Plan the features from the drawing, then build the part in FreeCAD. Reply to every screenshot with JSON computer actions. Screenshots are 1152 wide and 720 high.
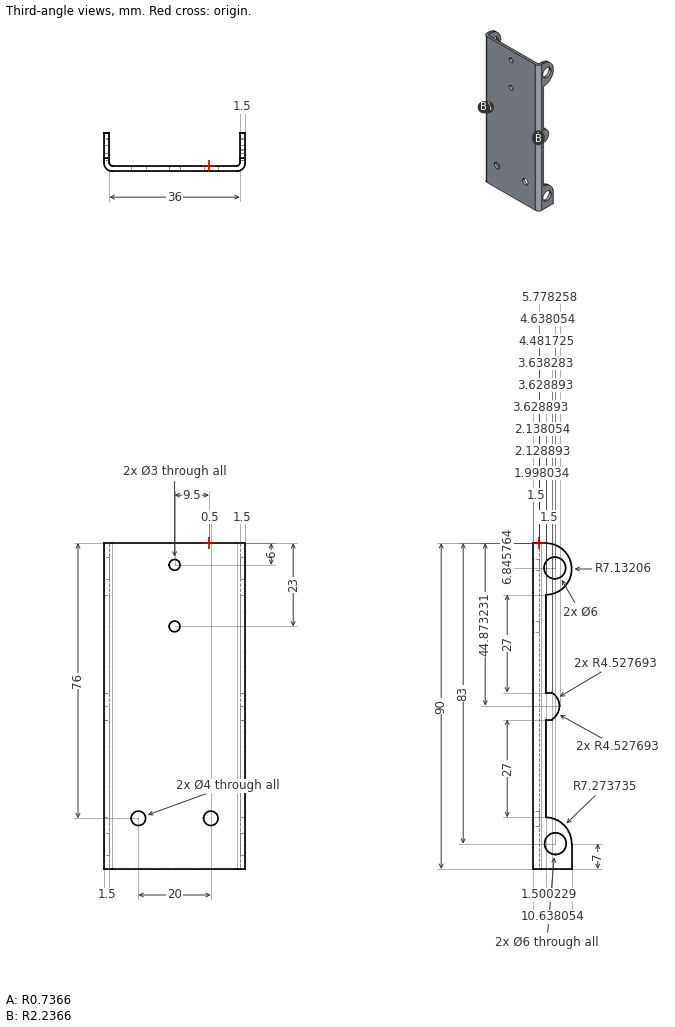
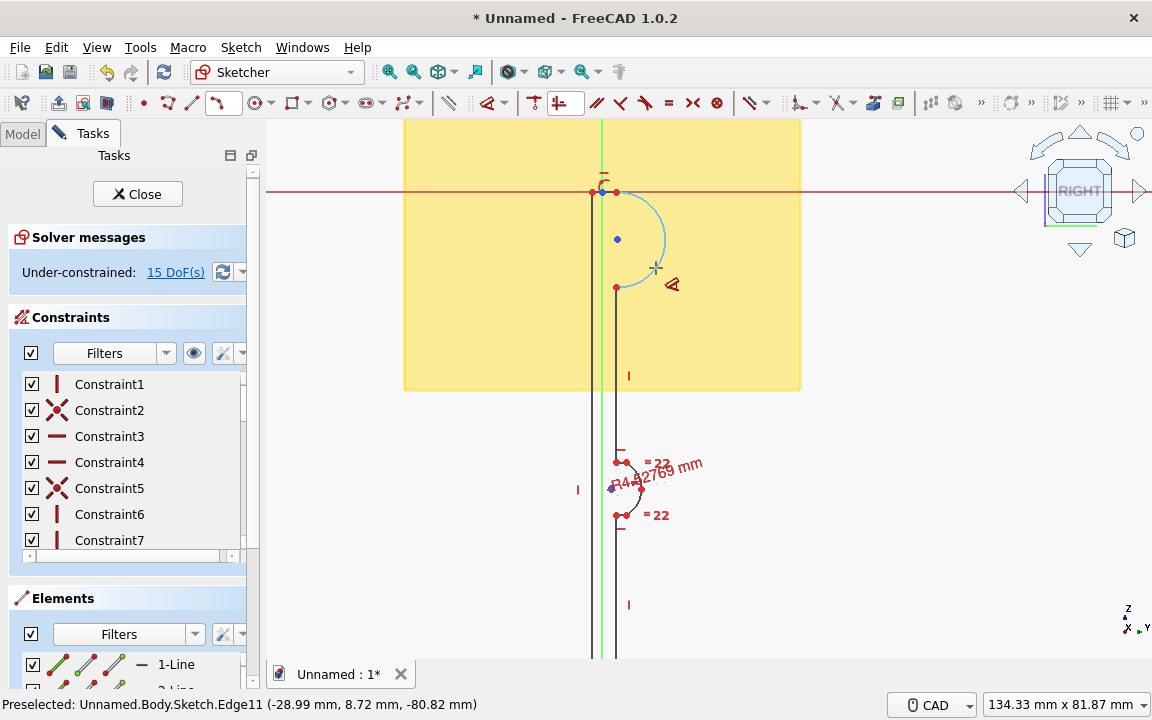
{"action": "left_click", "coordinate": [656, 268]}
{"action": "left_click", "coordinate": [682, 287]}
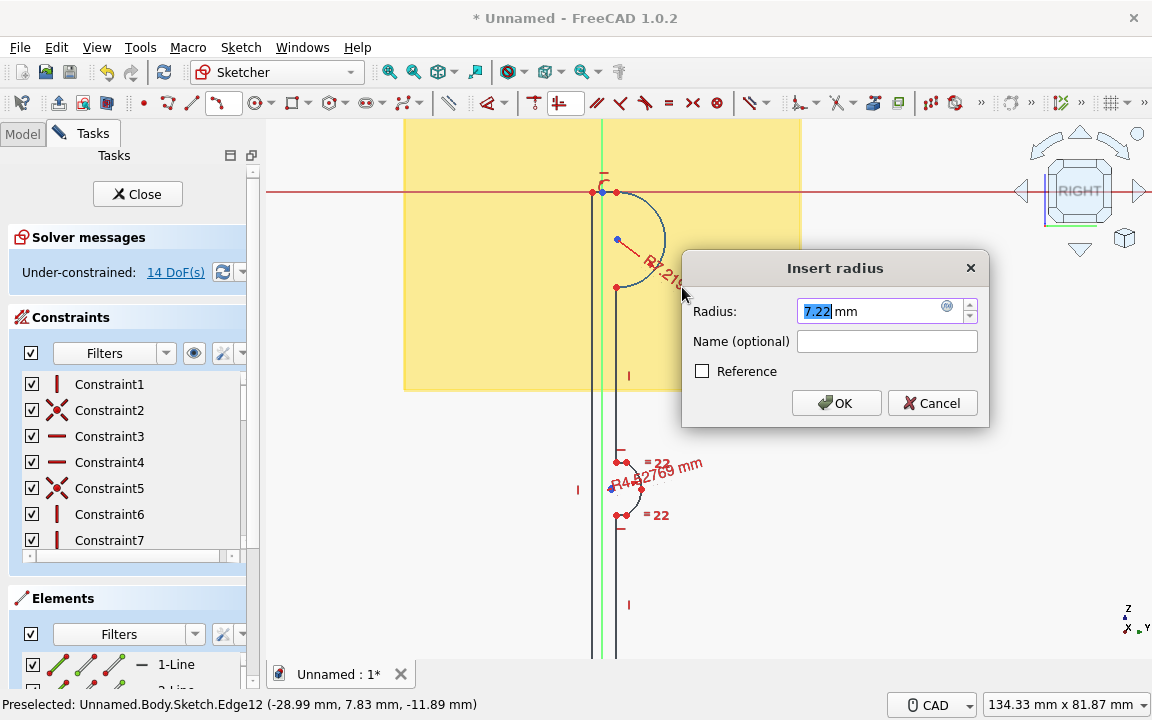
{"action": "type", "text": "7.13206"}
{"action": "key", "text": "Return"}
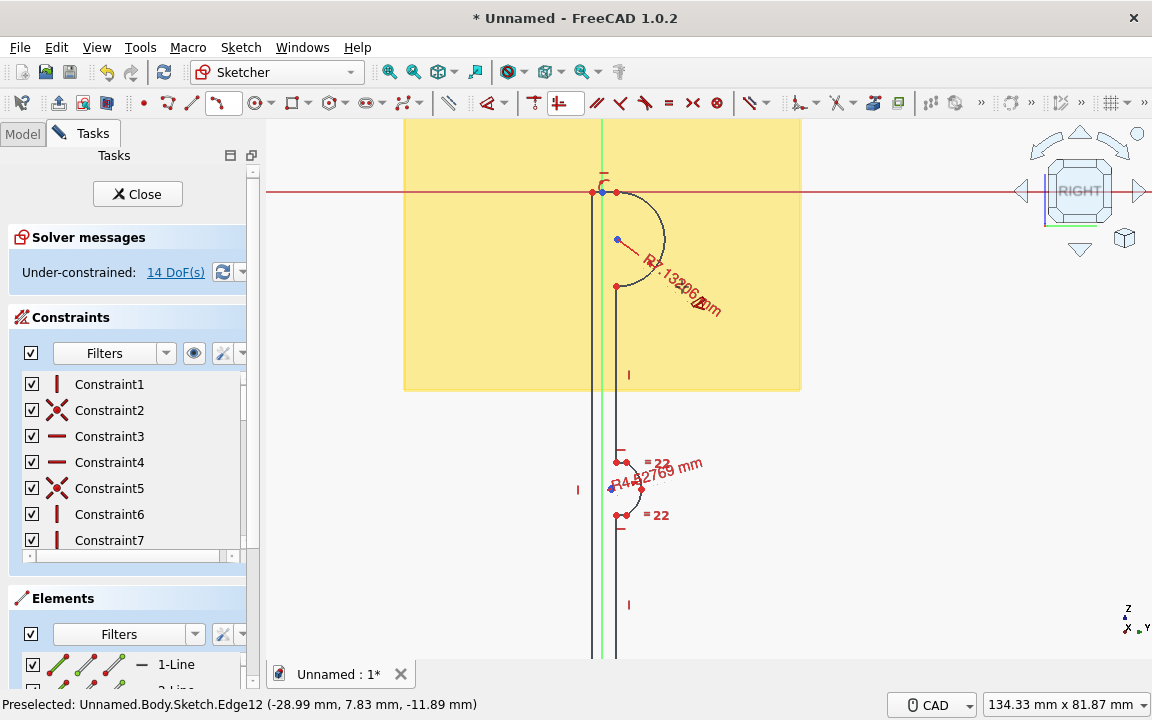
{"action": "scroll", "coordinate": [656, 267], "scroll_direction": "down", "scroll_amount": 3}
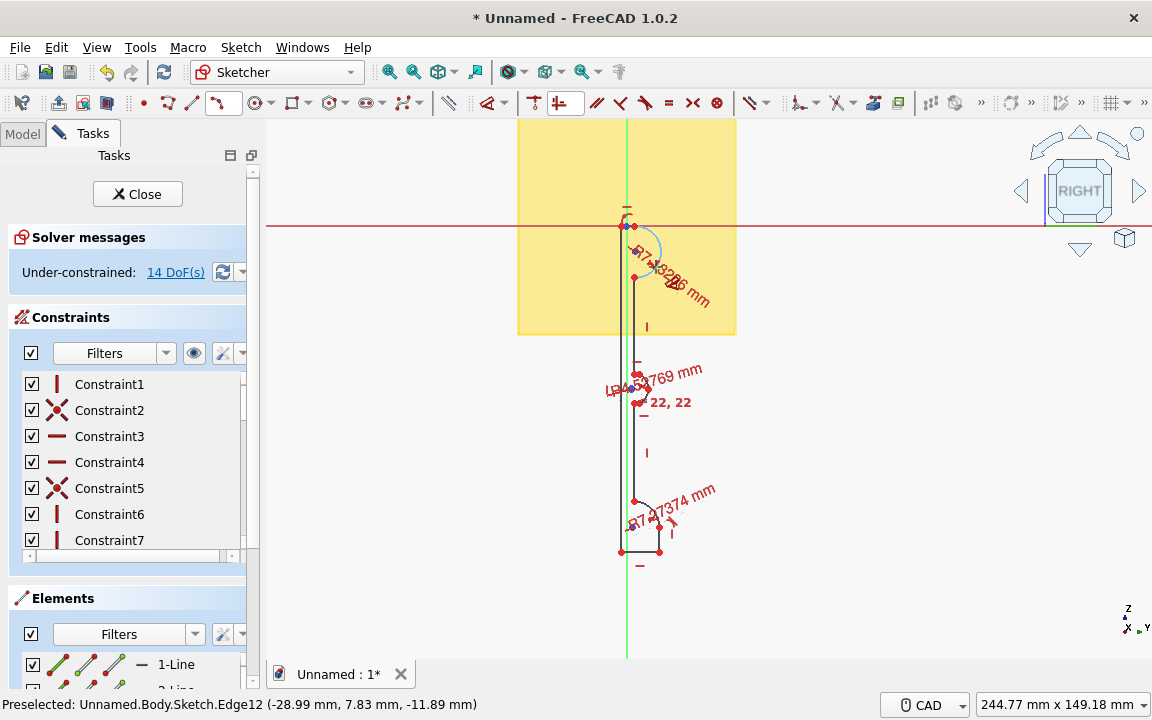
{"action": "scroll", "coordinate": [659, 535], "scroll_direction": "up", "scroll_amount": 4}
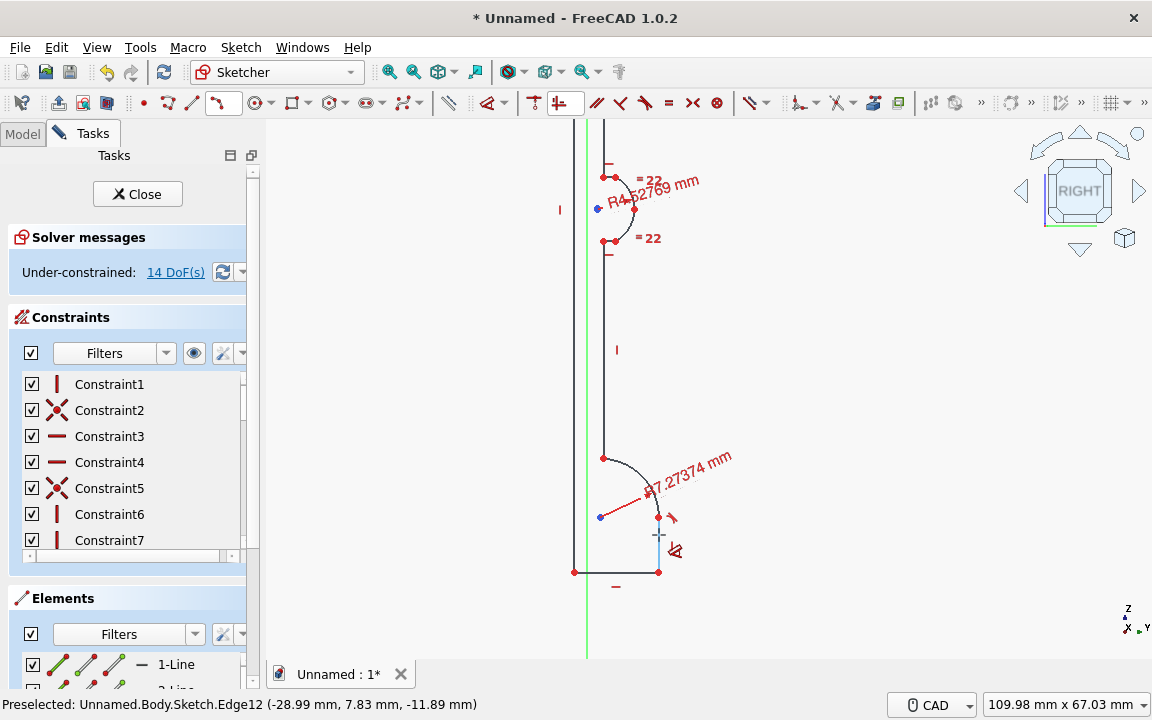
{"action": "left_click", "coordinate": [659, 534]}
{"action": "left_click", "coordinate": [693, 545]}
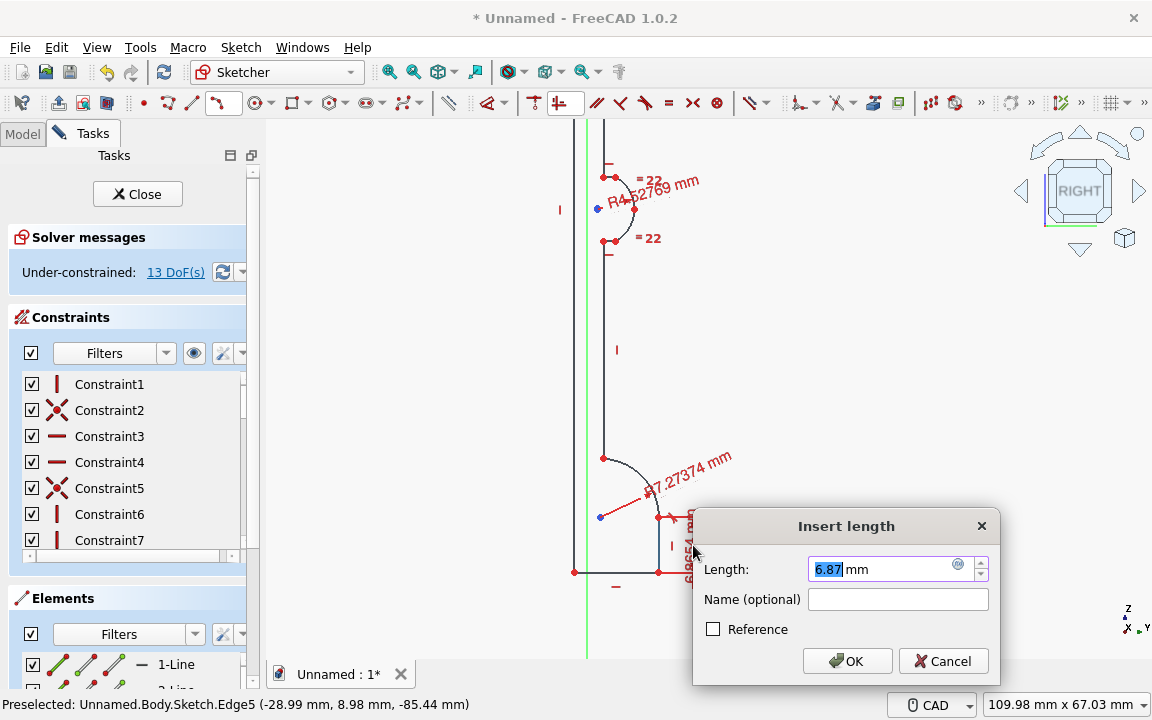
{"action": "type", "text": "7"}
{"action": "key", "text": "Return"}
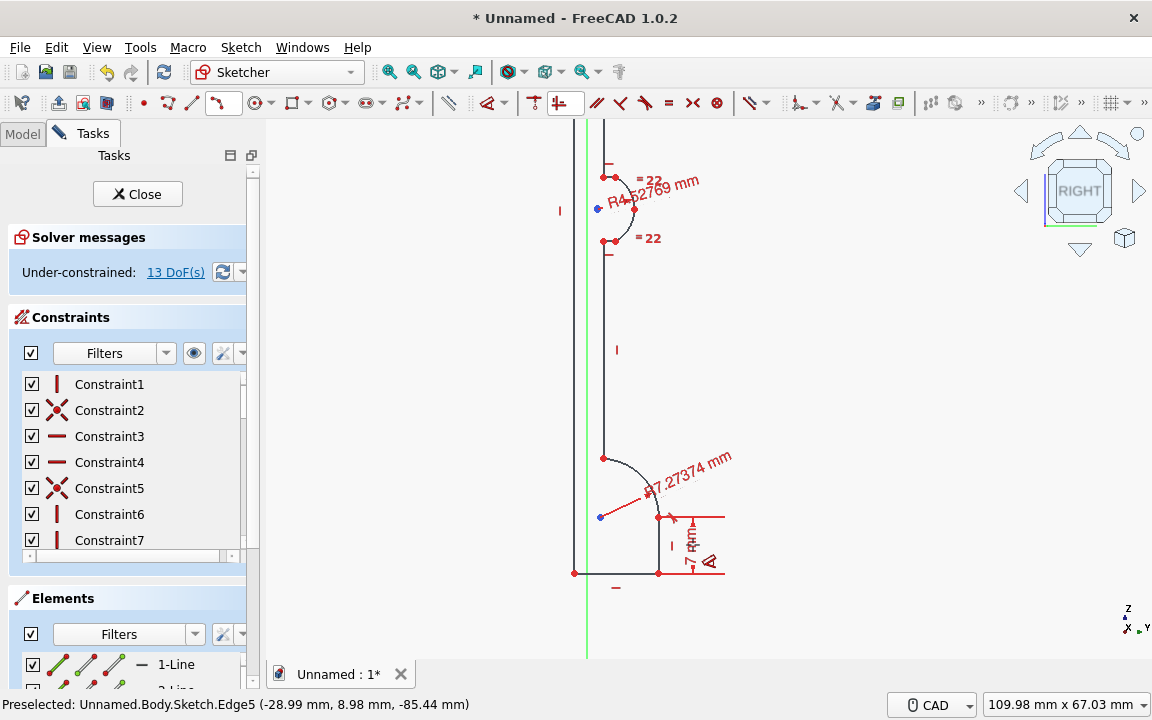
{"action": "scroll", "coordinate": [659, 536], "scroll_direction": "down", "scroll_amount": 4}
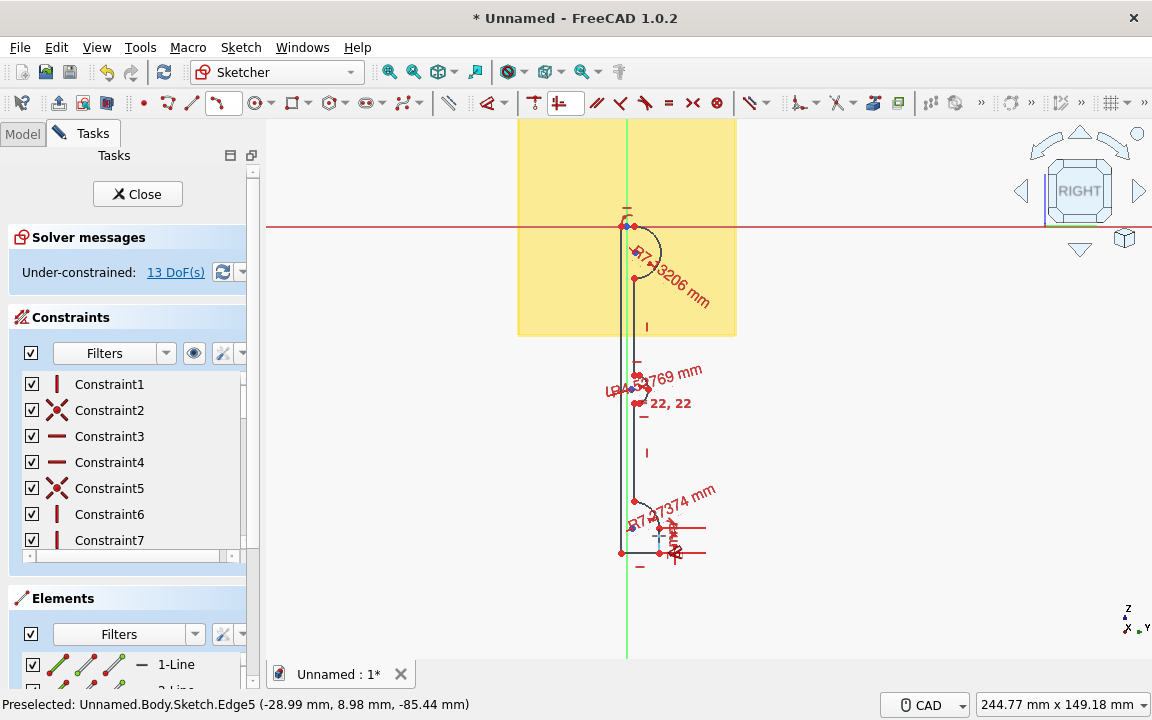
{"action": "scroll", "coordinate": [634, 307], "scroll_direction": "up", "scroll_amount": 3}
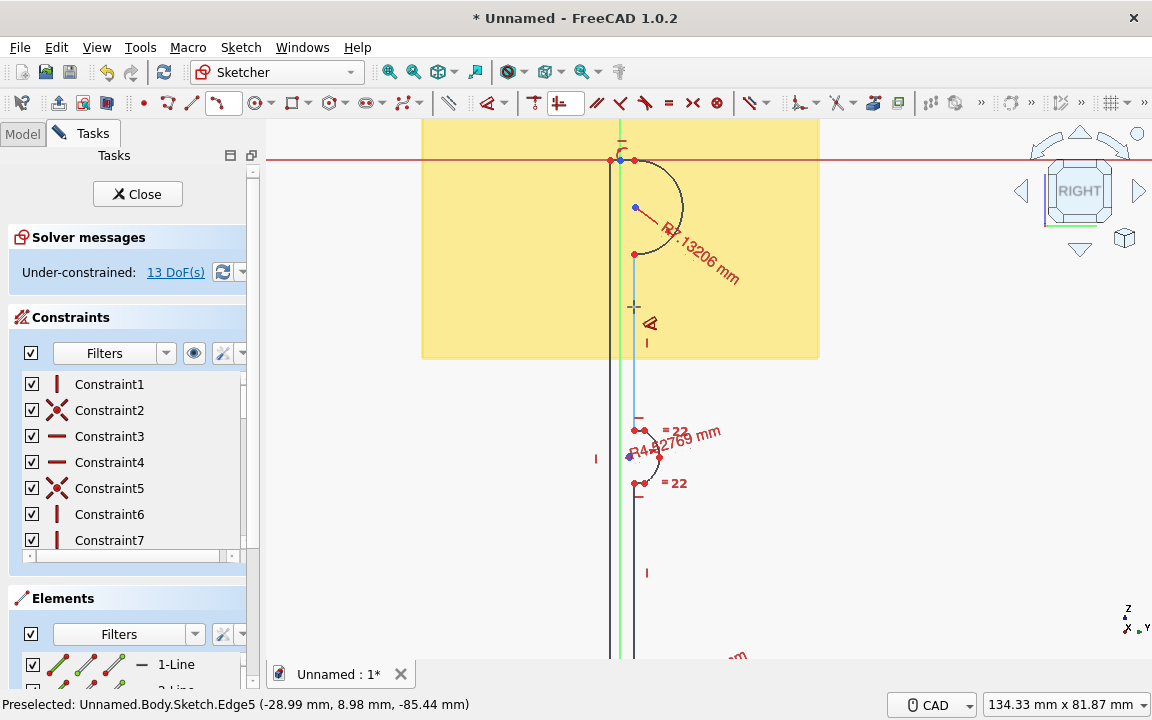
{"action": "left_click", "coordinate": [634, 307]}
{"action": "left_click", "coordinate": [668, 343]}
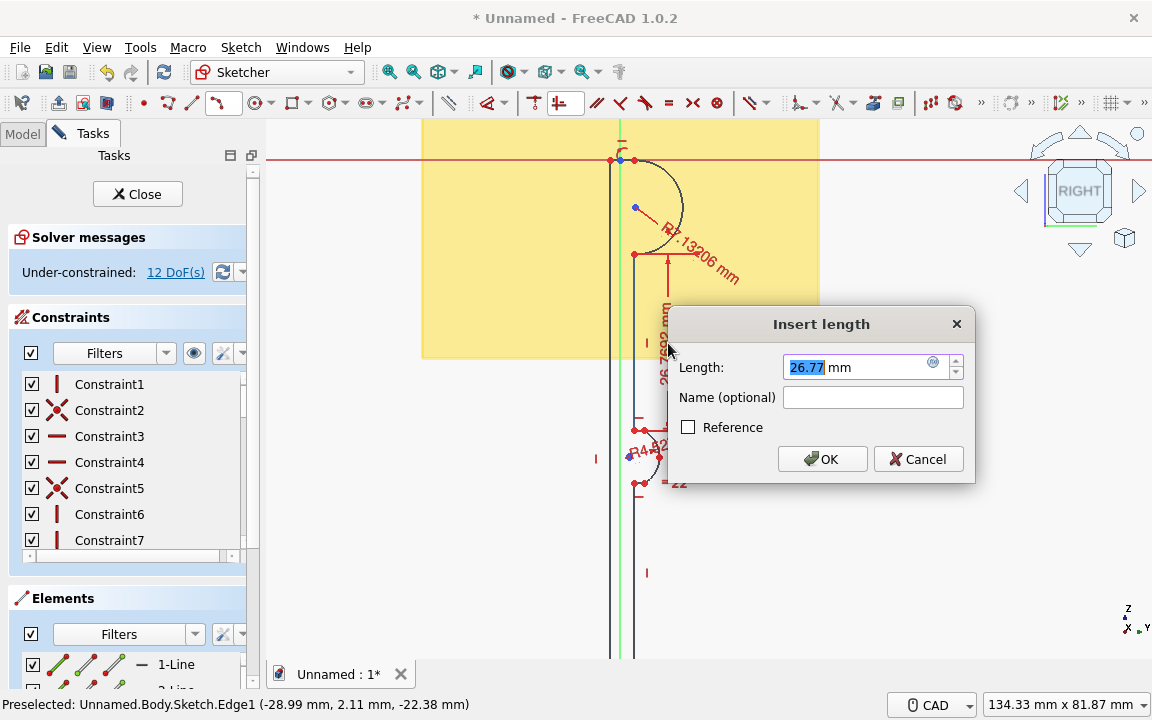
{"action": "type", "text": "27"}
{"action": "key", "text": "Return"}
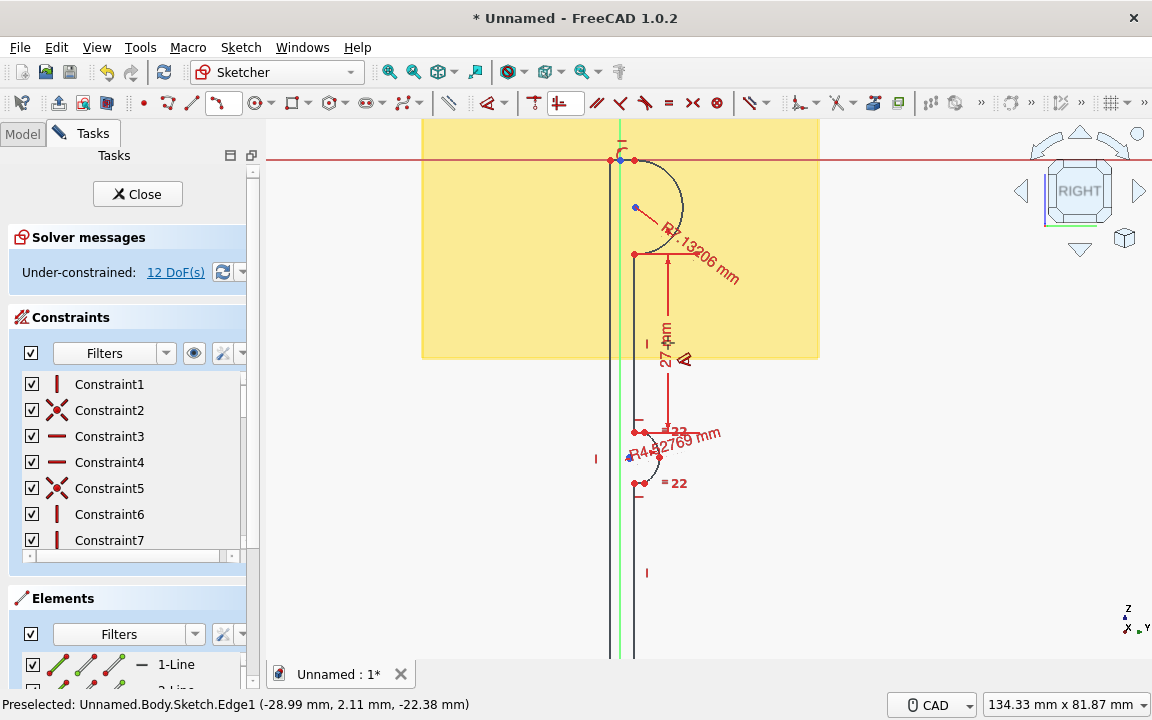
{"action": "left_click", "coordinate": [634, 537]}
{"action": "left_click", "coordinate": [668, 557]}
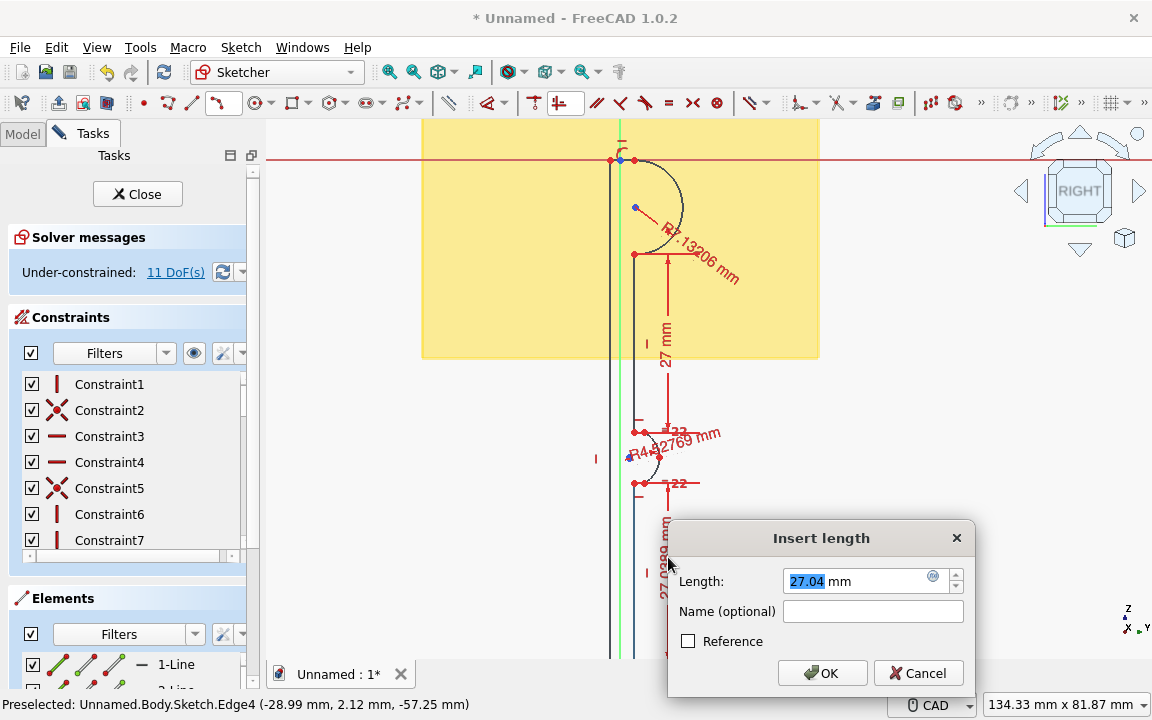
{"action": "type", "text": "27"}
{"action": "key", "text": "Return"}